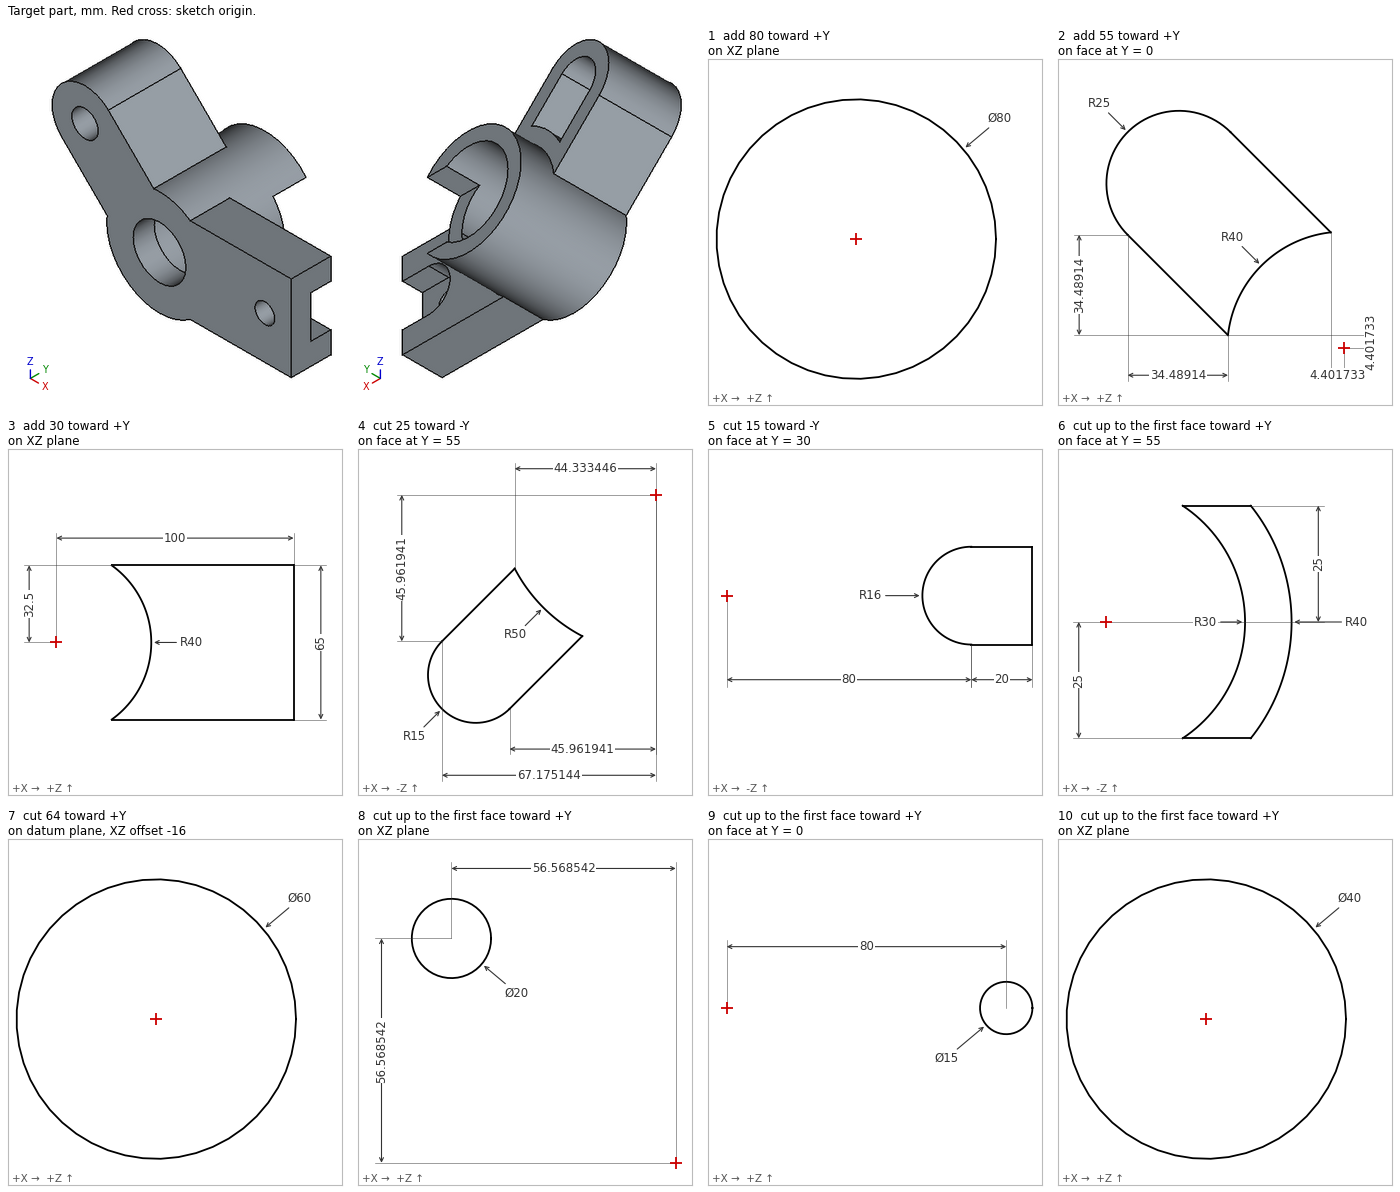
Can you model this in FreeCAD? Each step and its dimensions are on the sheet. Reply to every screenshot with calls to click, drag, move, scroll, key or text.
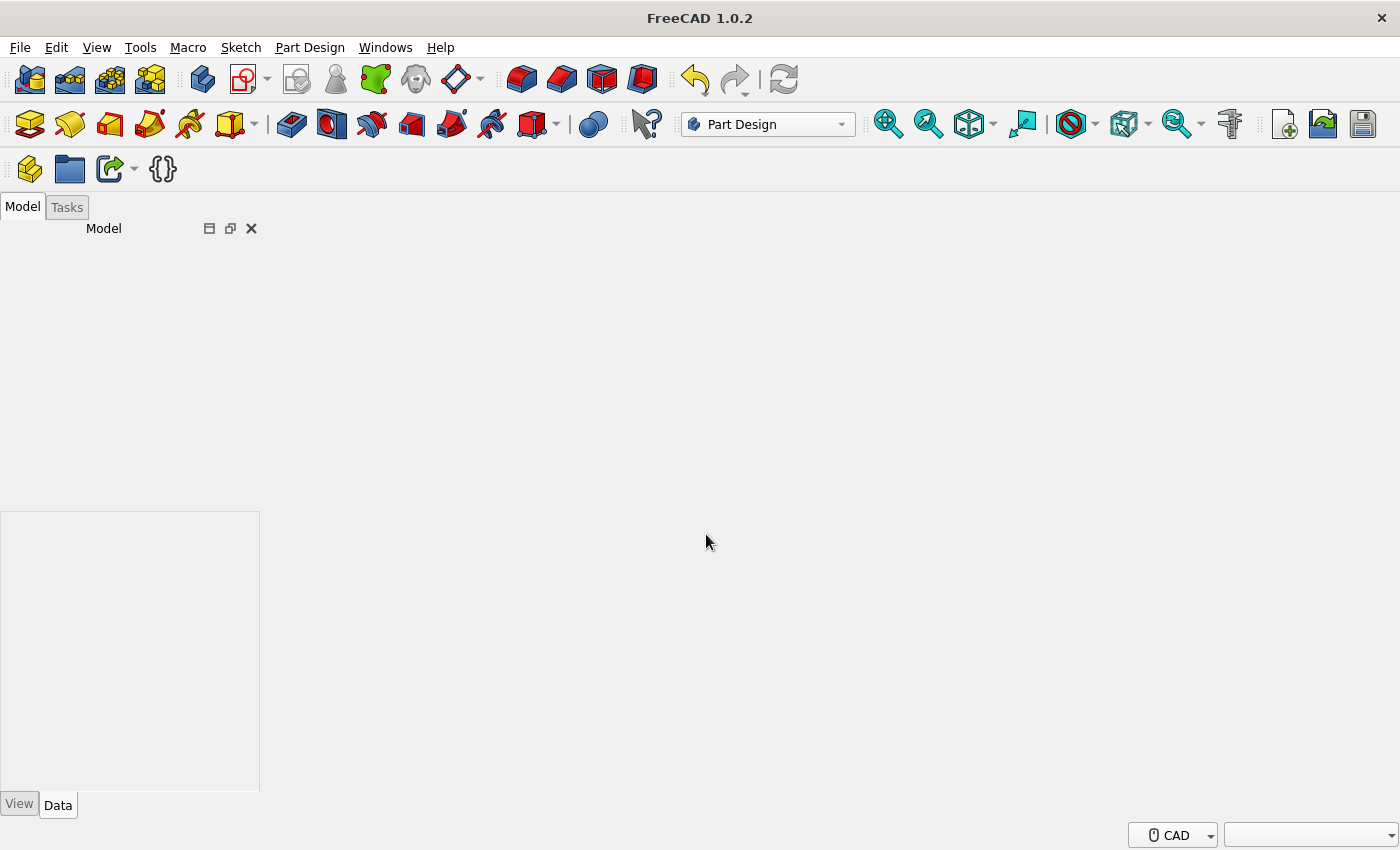
click(1284, 124)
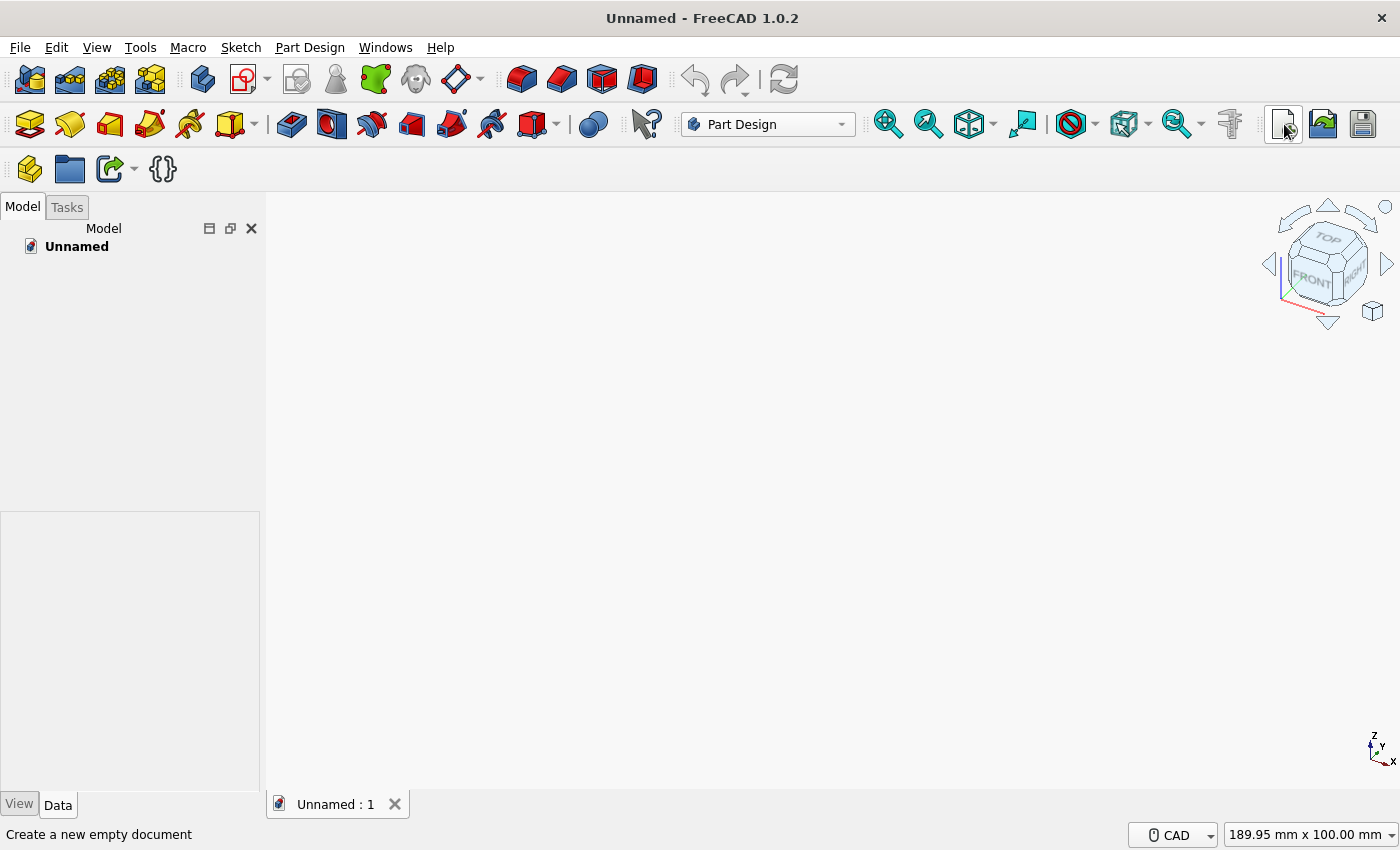
click(244, 80)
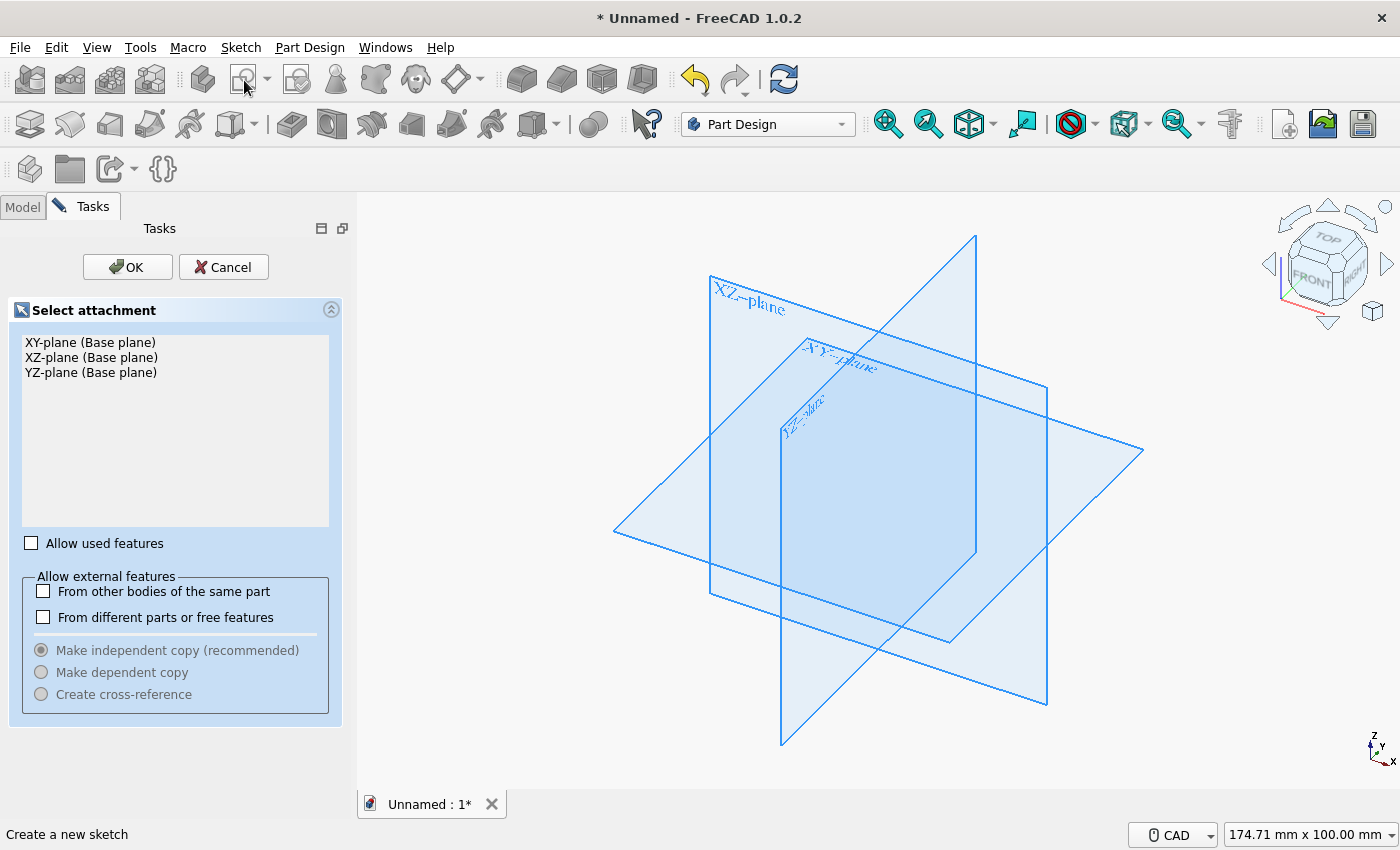
click(82, 358)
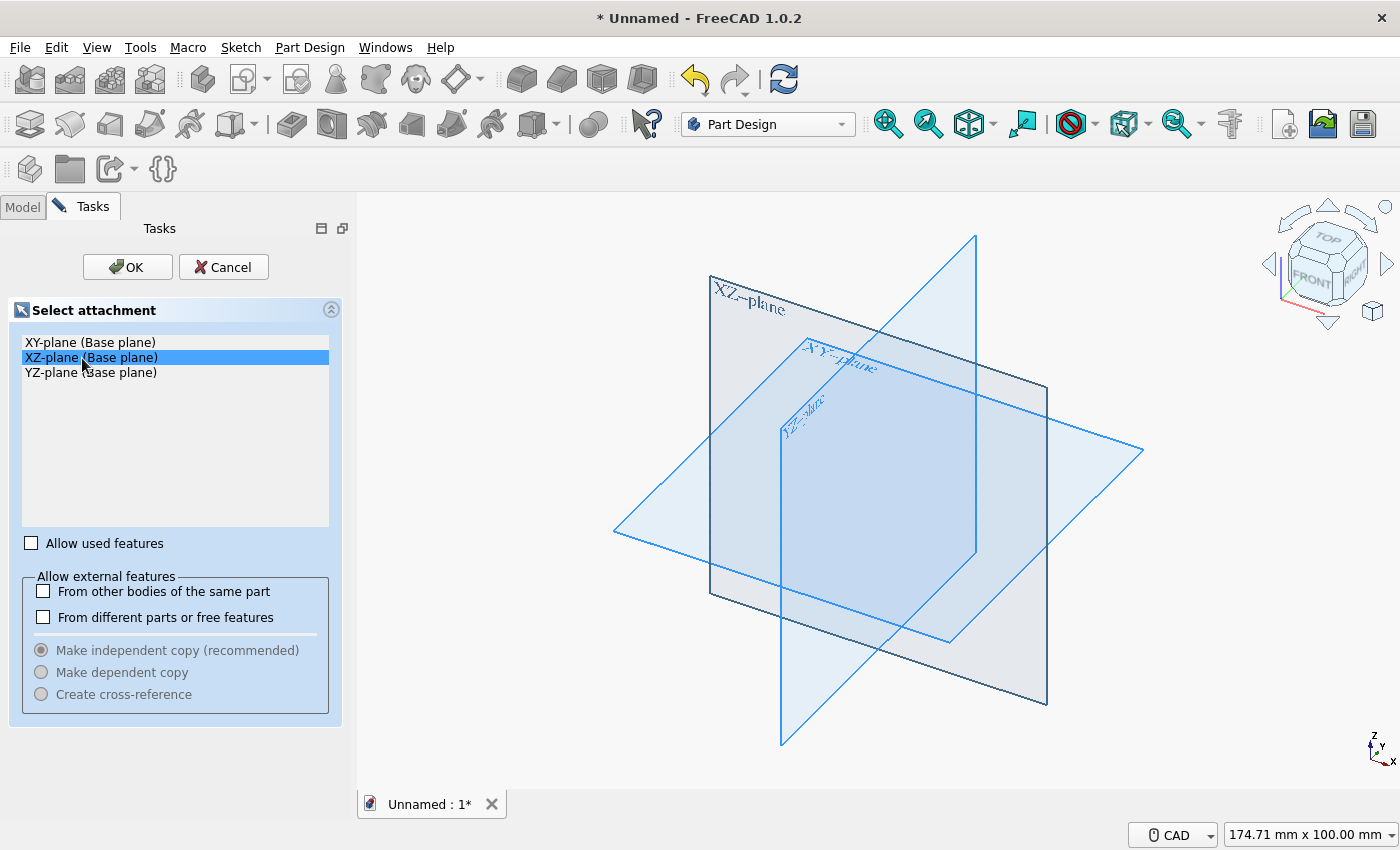
click(128, 267)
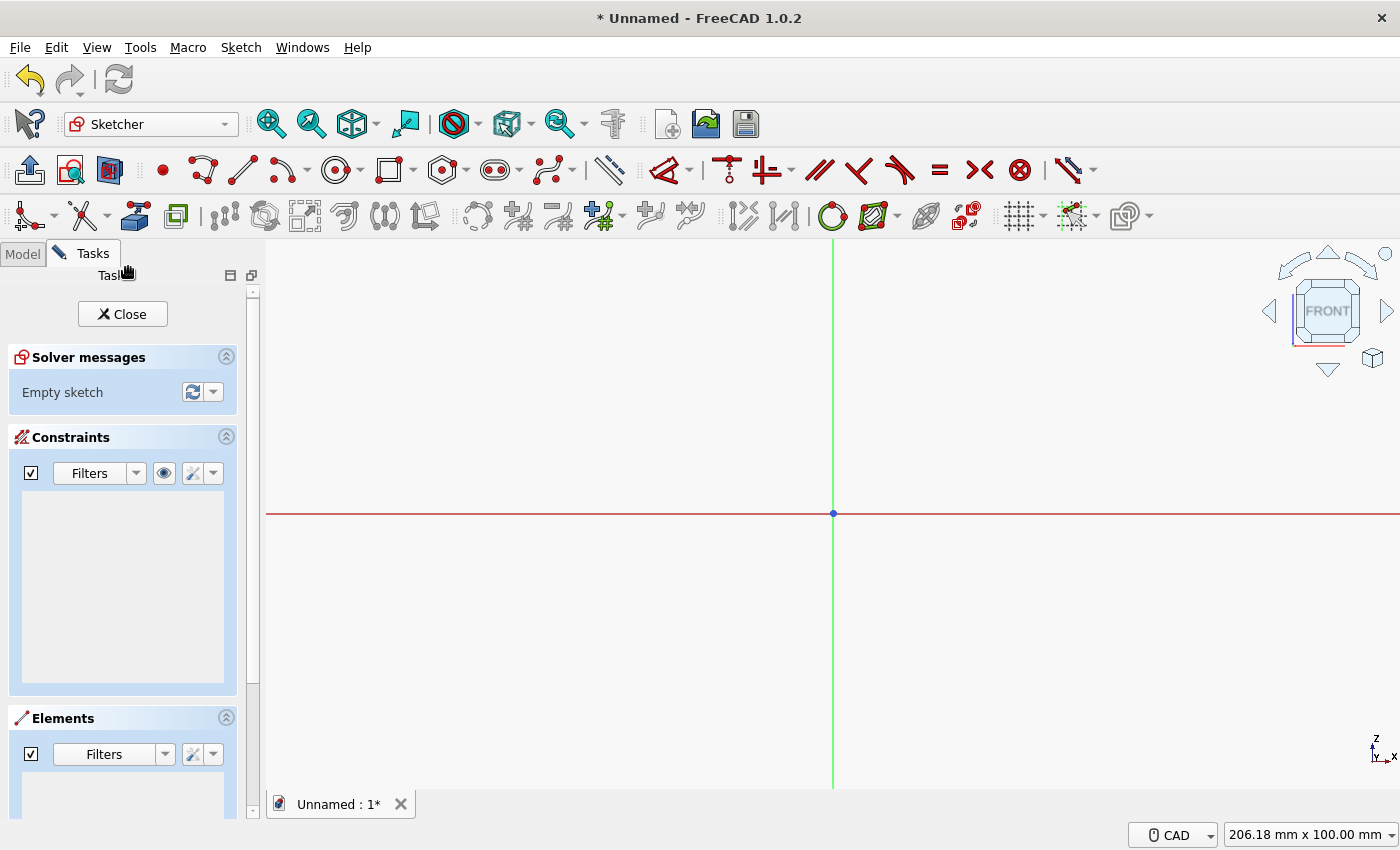
click(336, 170)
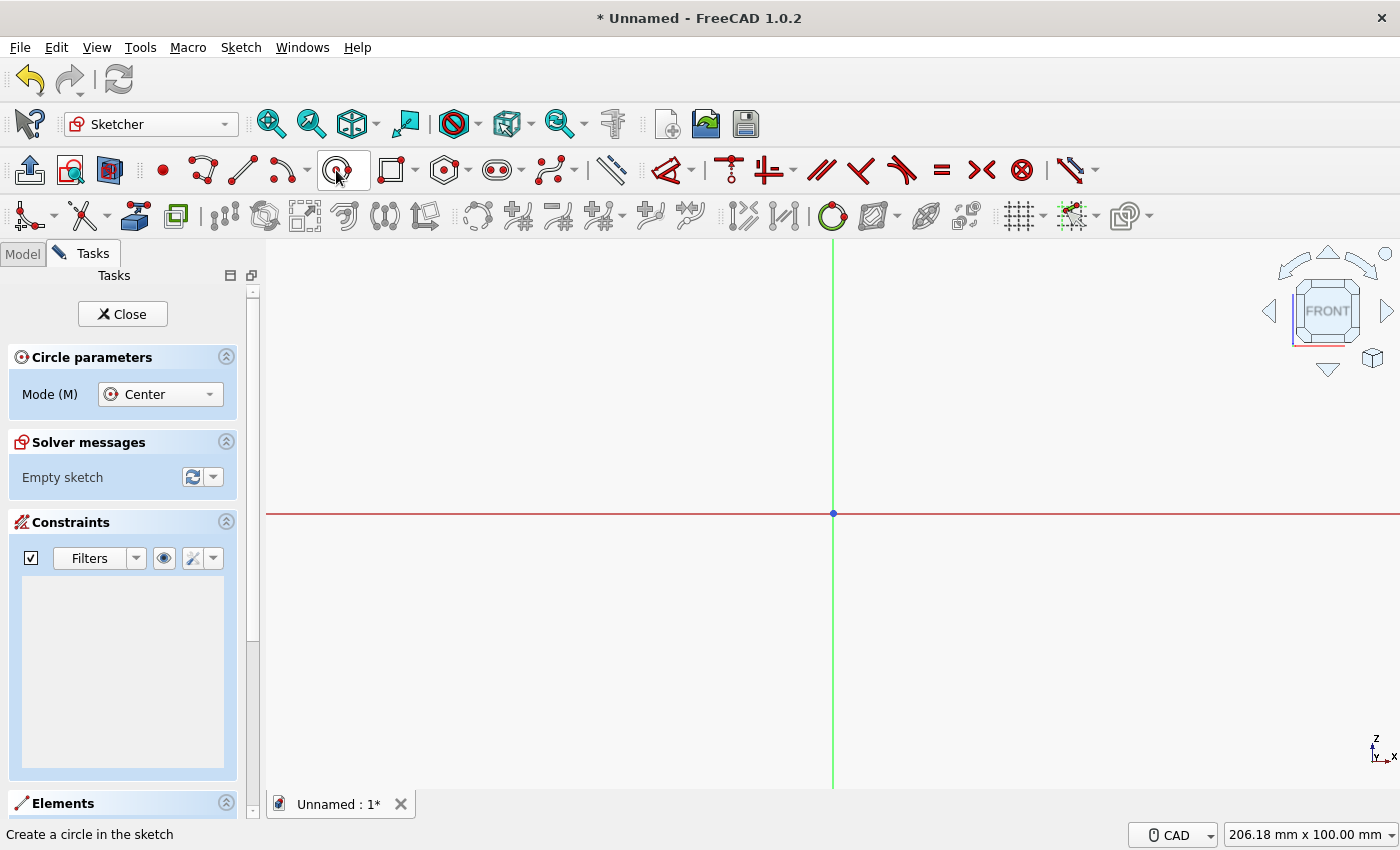
click(833, 514)
click(989, 358)
key(Escape)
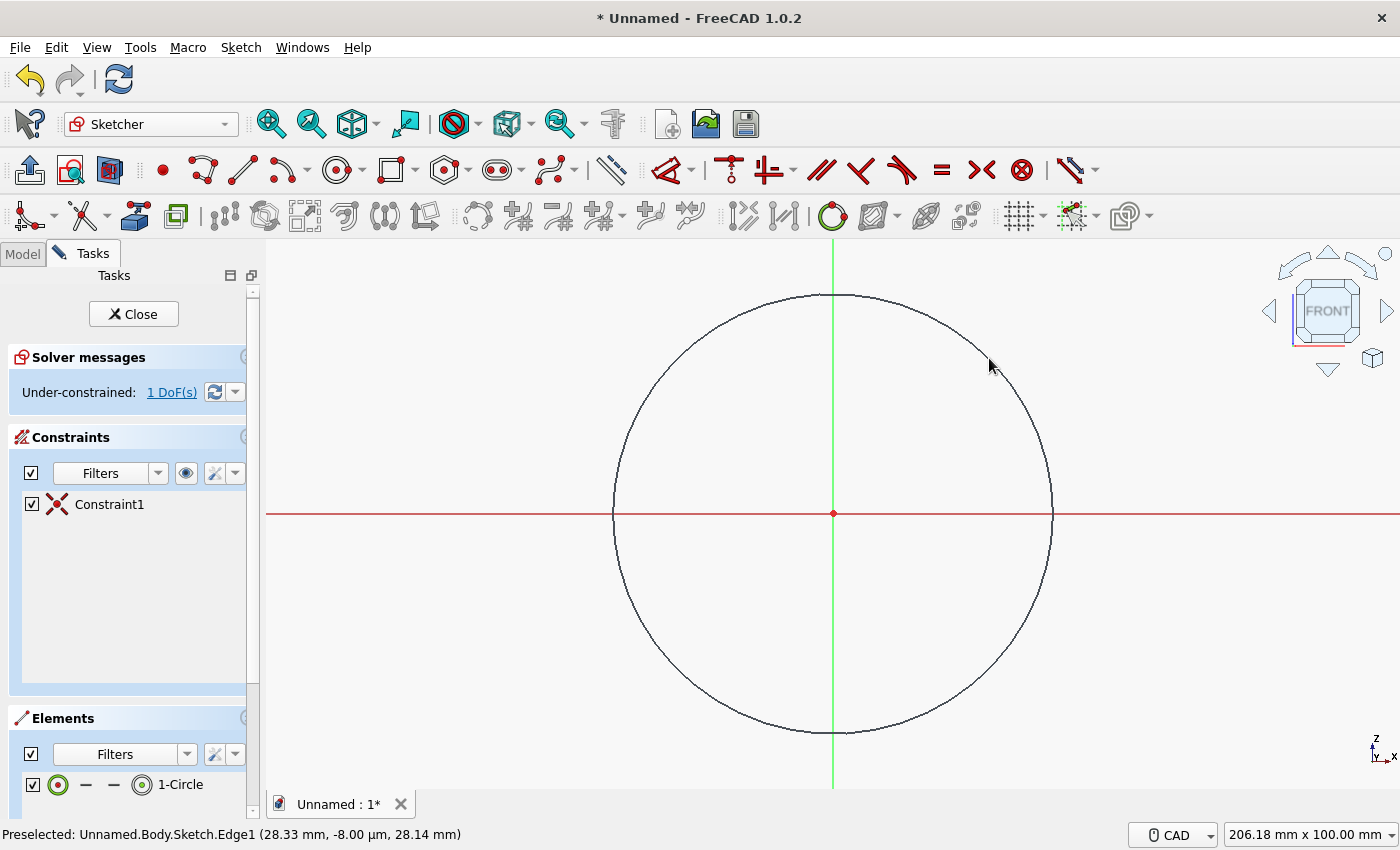
click(988, 358)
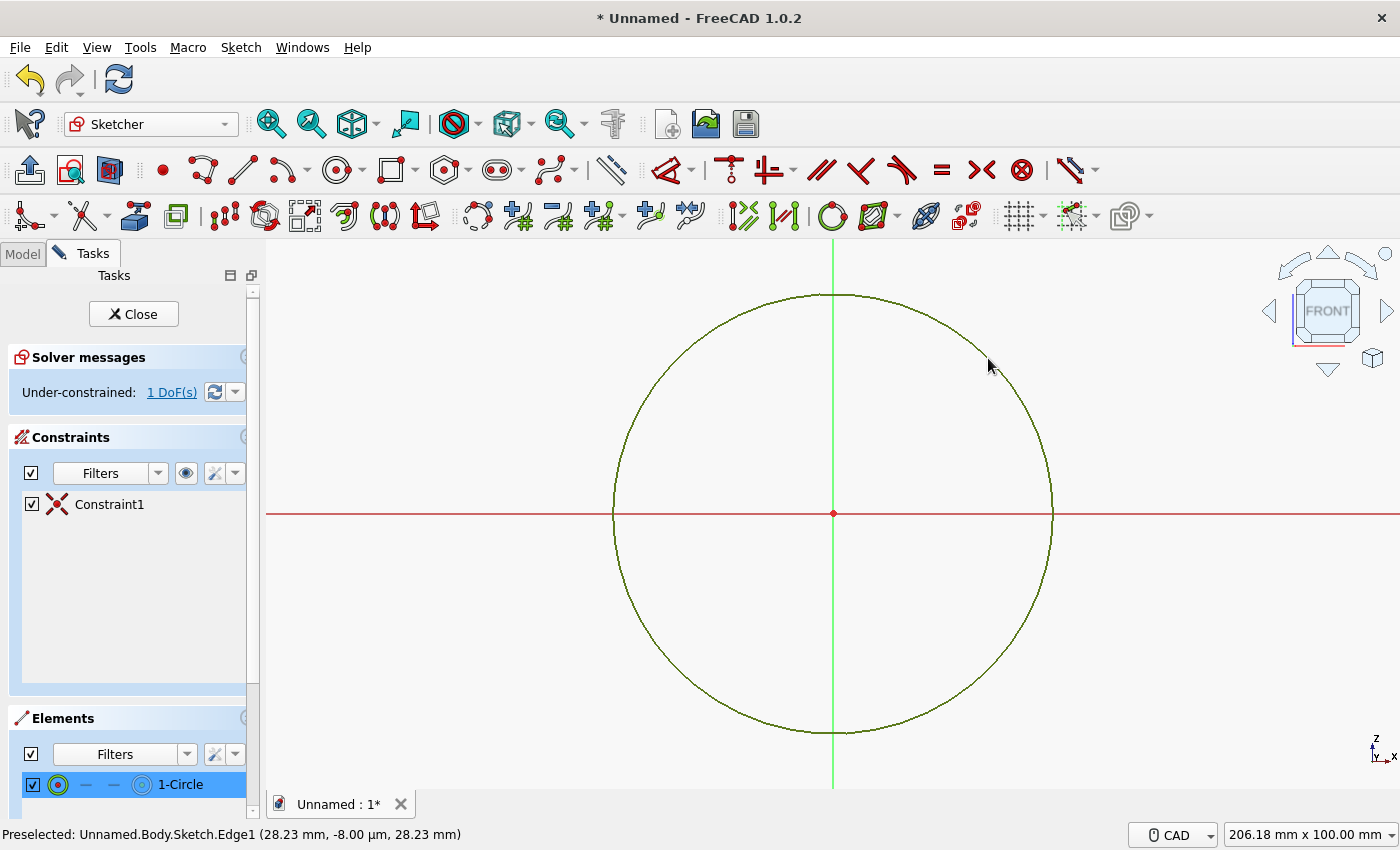
click(694, 170)